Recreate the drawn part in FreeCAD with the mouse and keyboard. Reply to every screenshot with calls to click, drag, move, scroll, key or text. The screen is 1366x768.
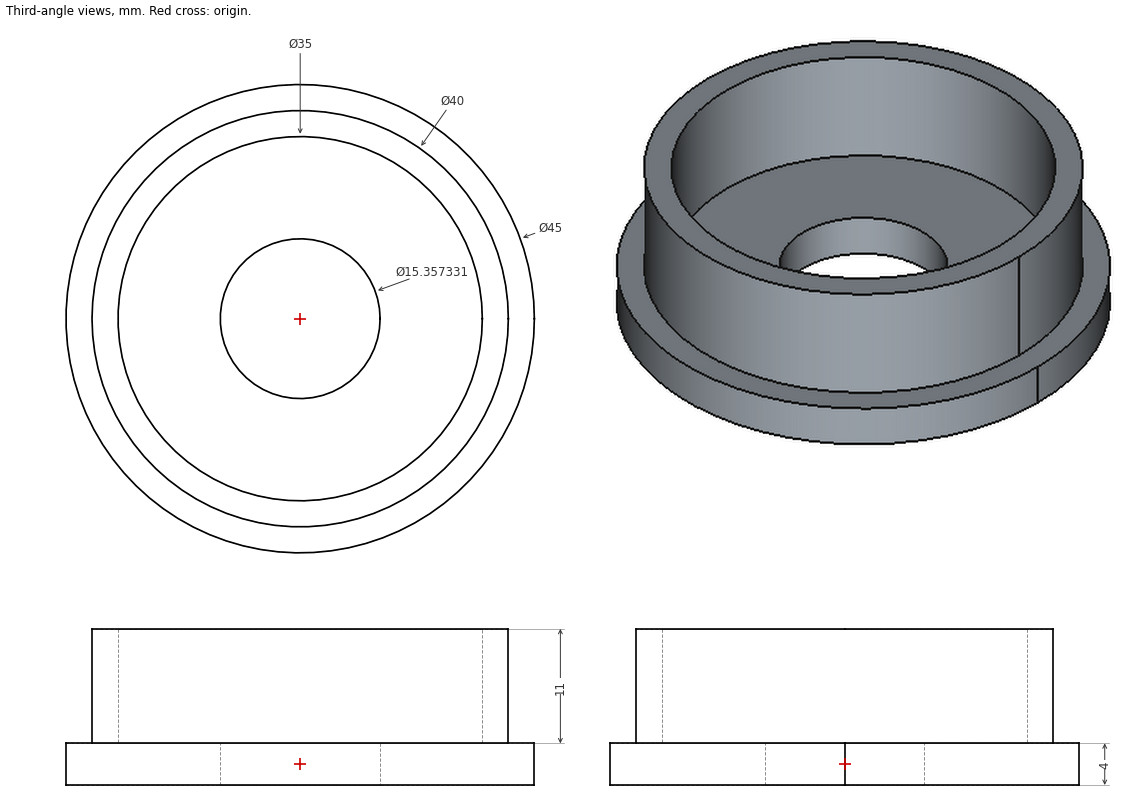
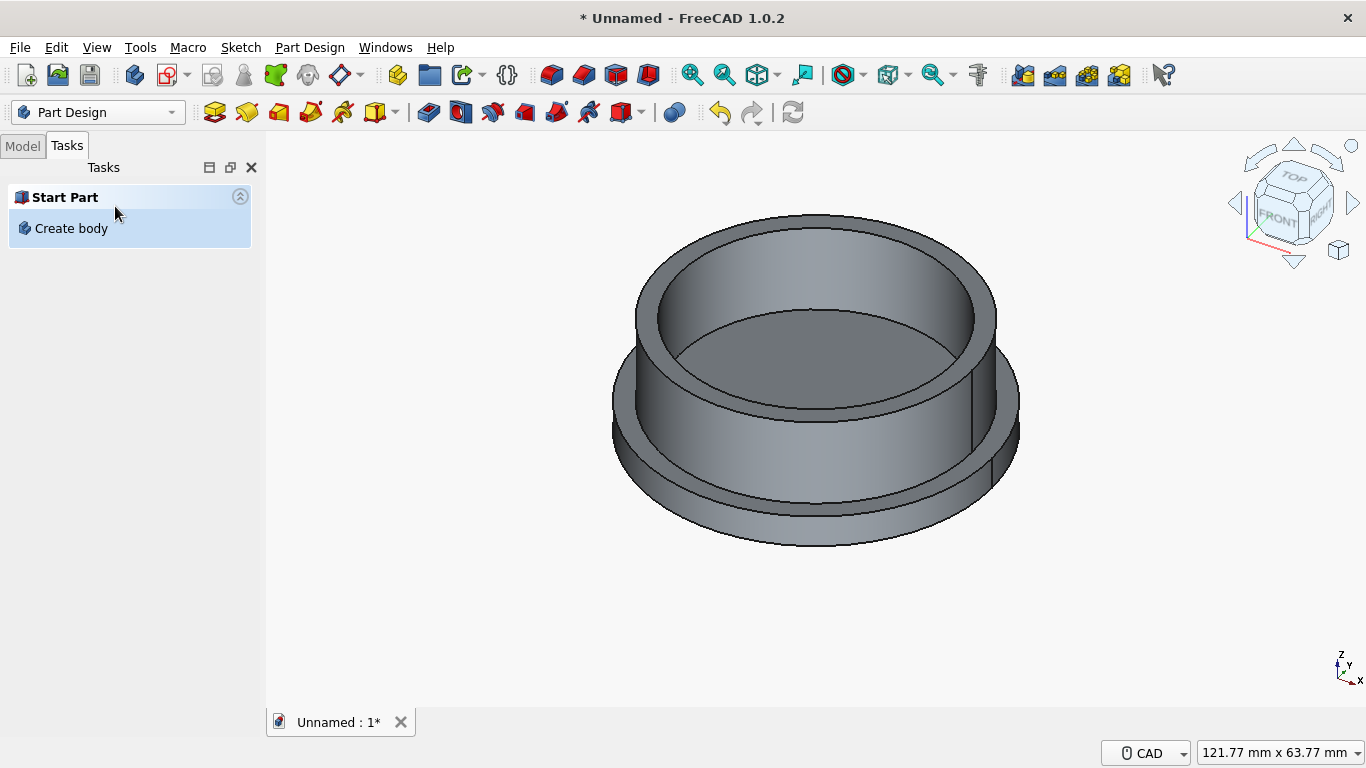
click(816, 399)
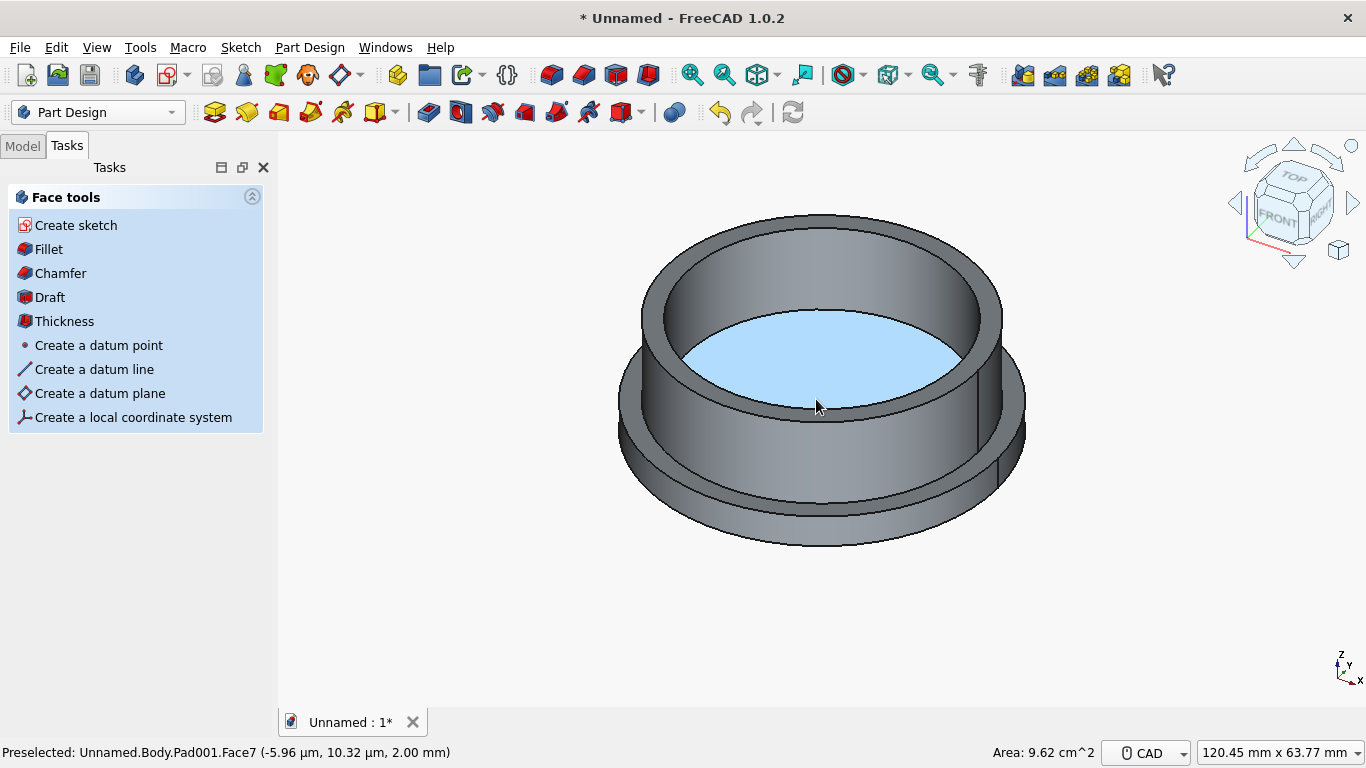
click(168, 76)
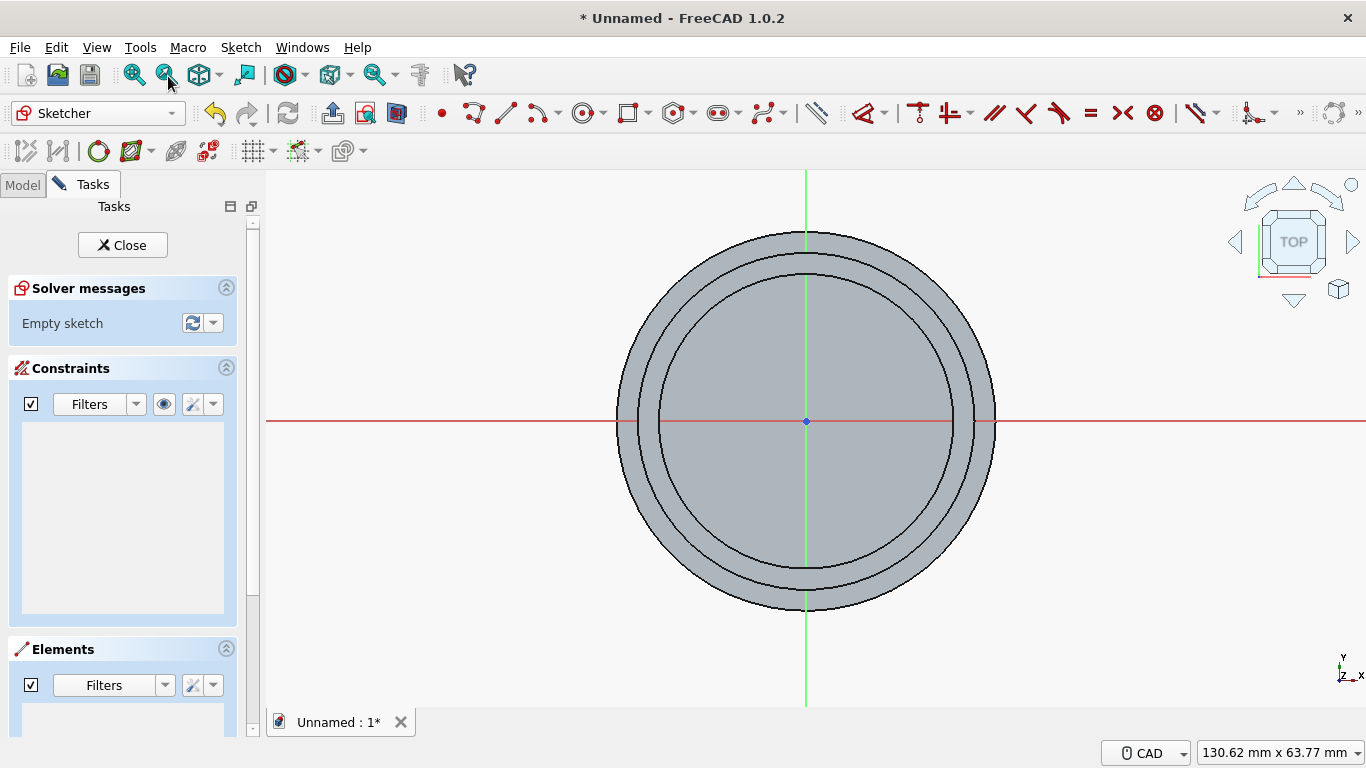
click(398, 114)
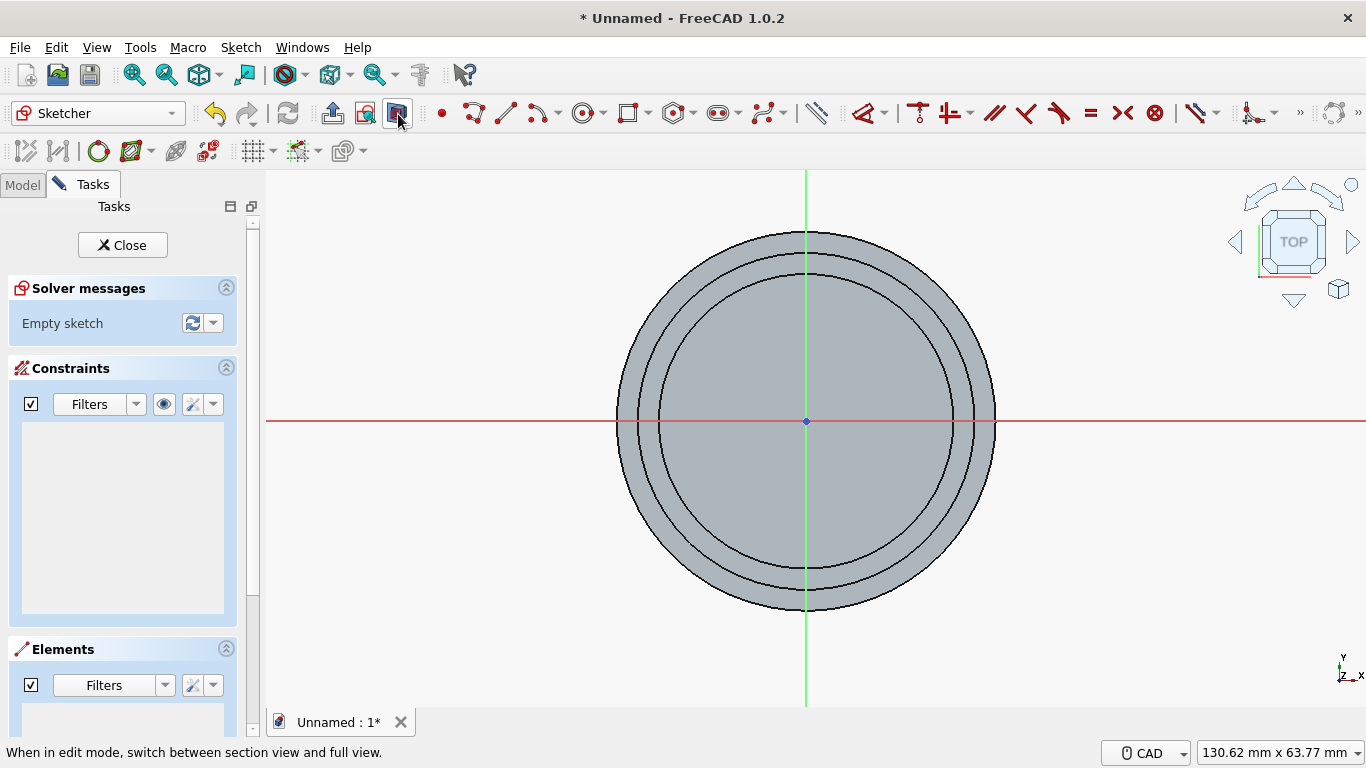
scroll(840, 411, up, 5)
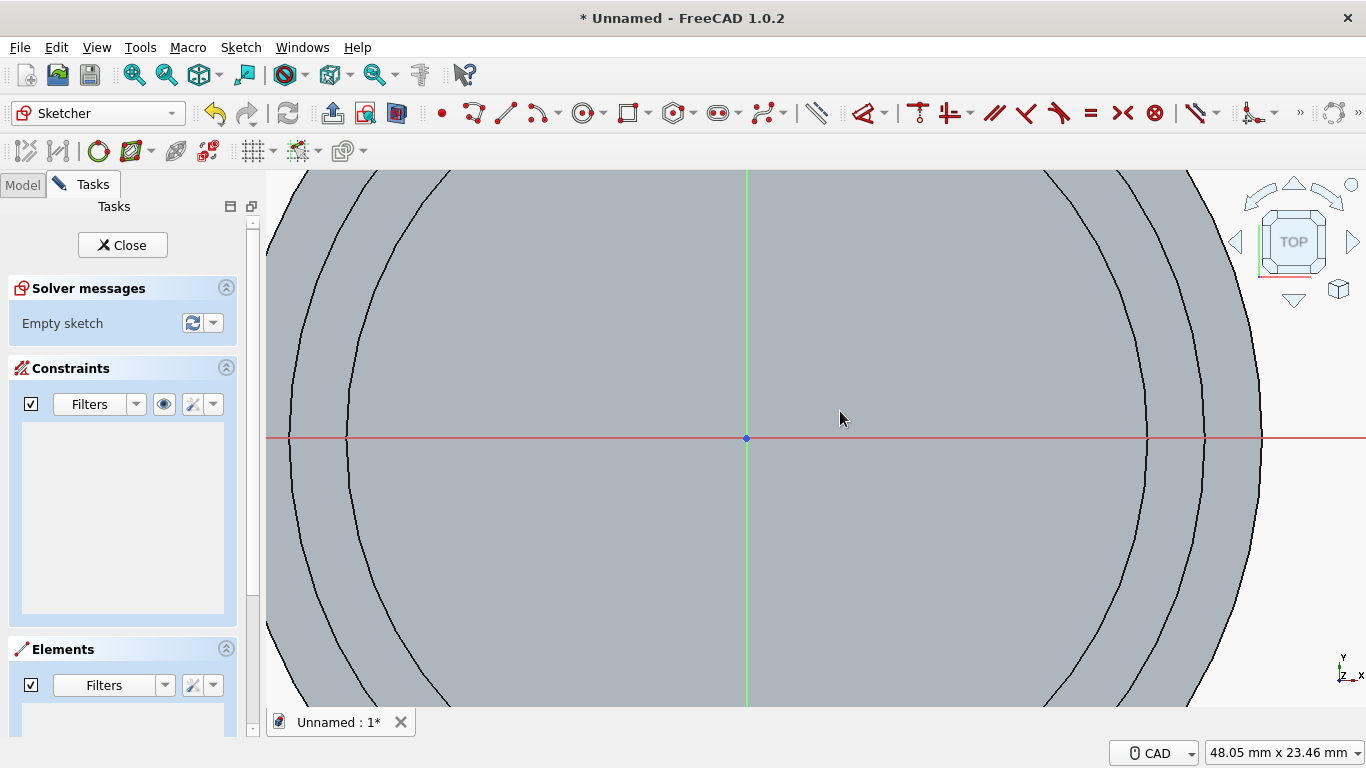
key(g)
key(c)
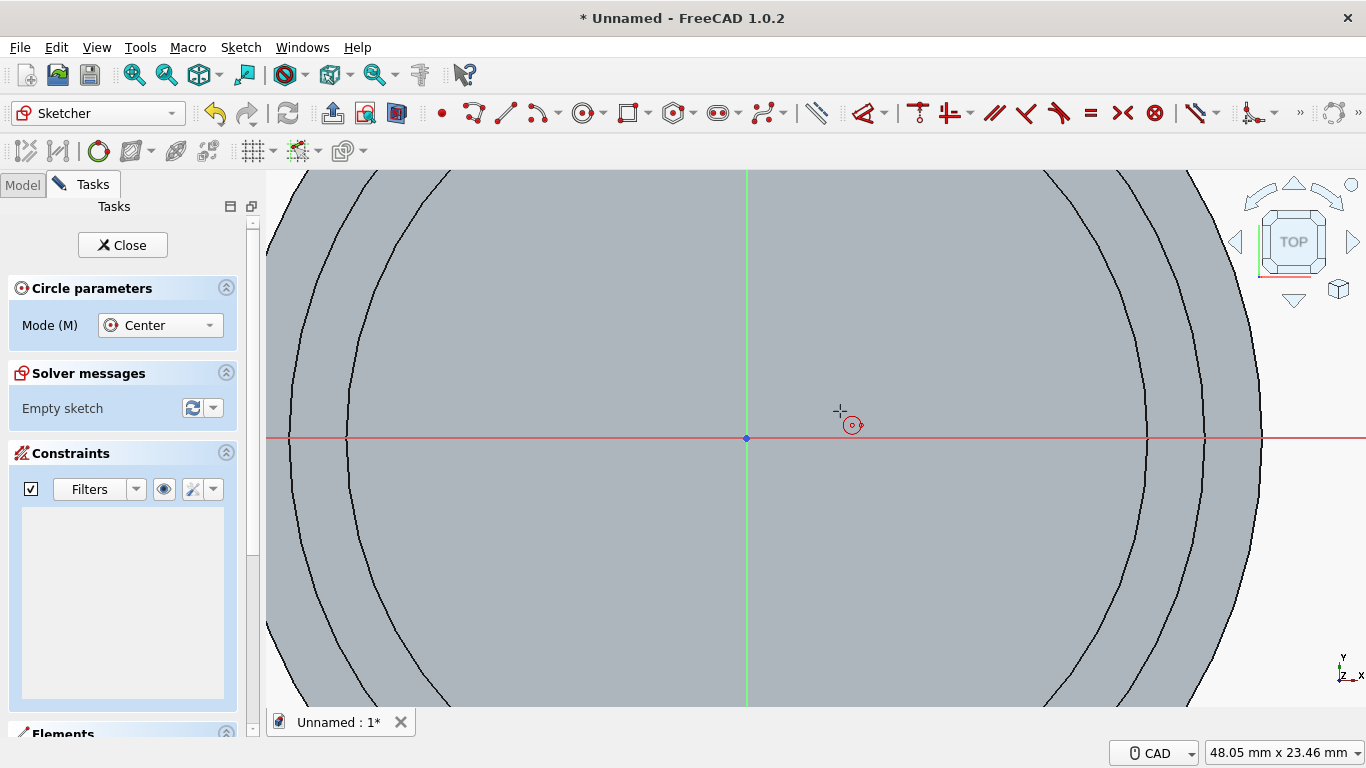
click(747, 438)
click(871, 314)
key(Escape)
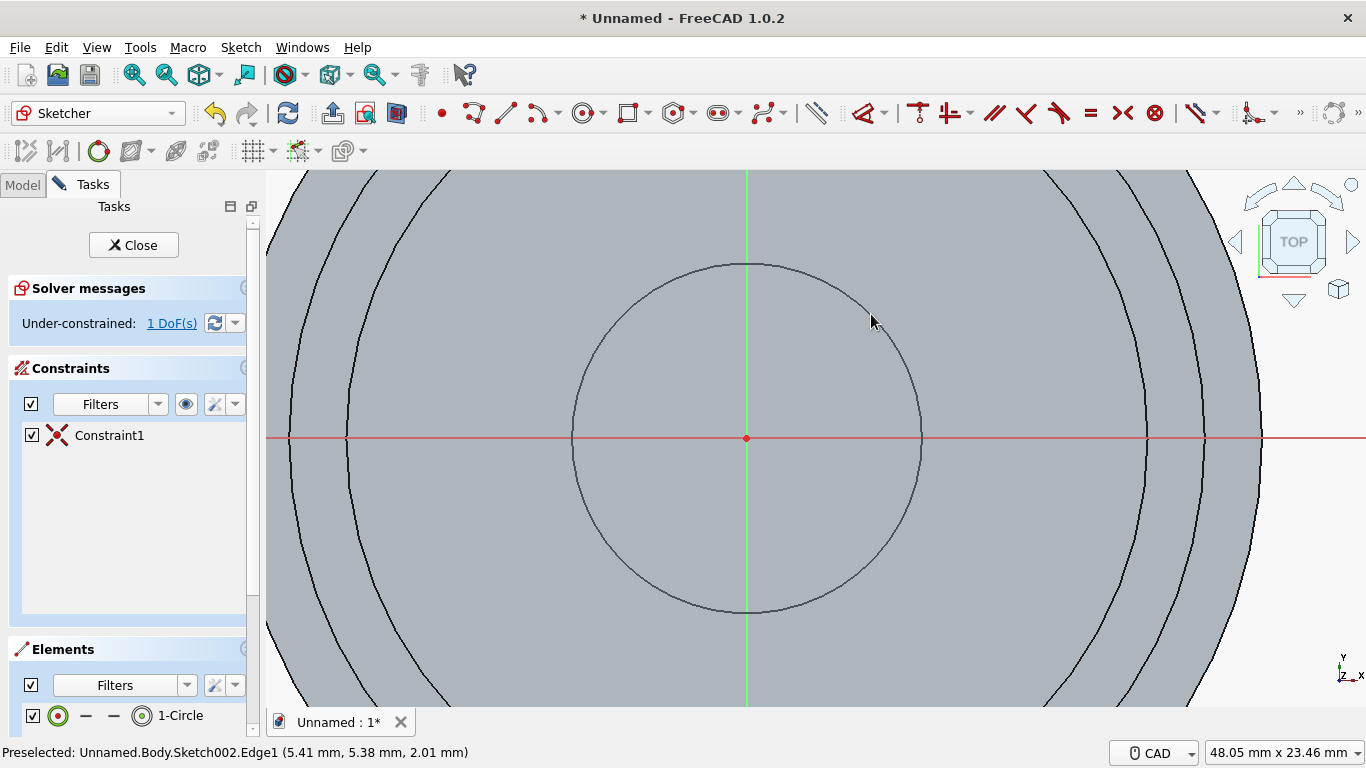
key(d)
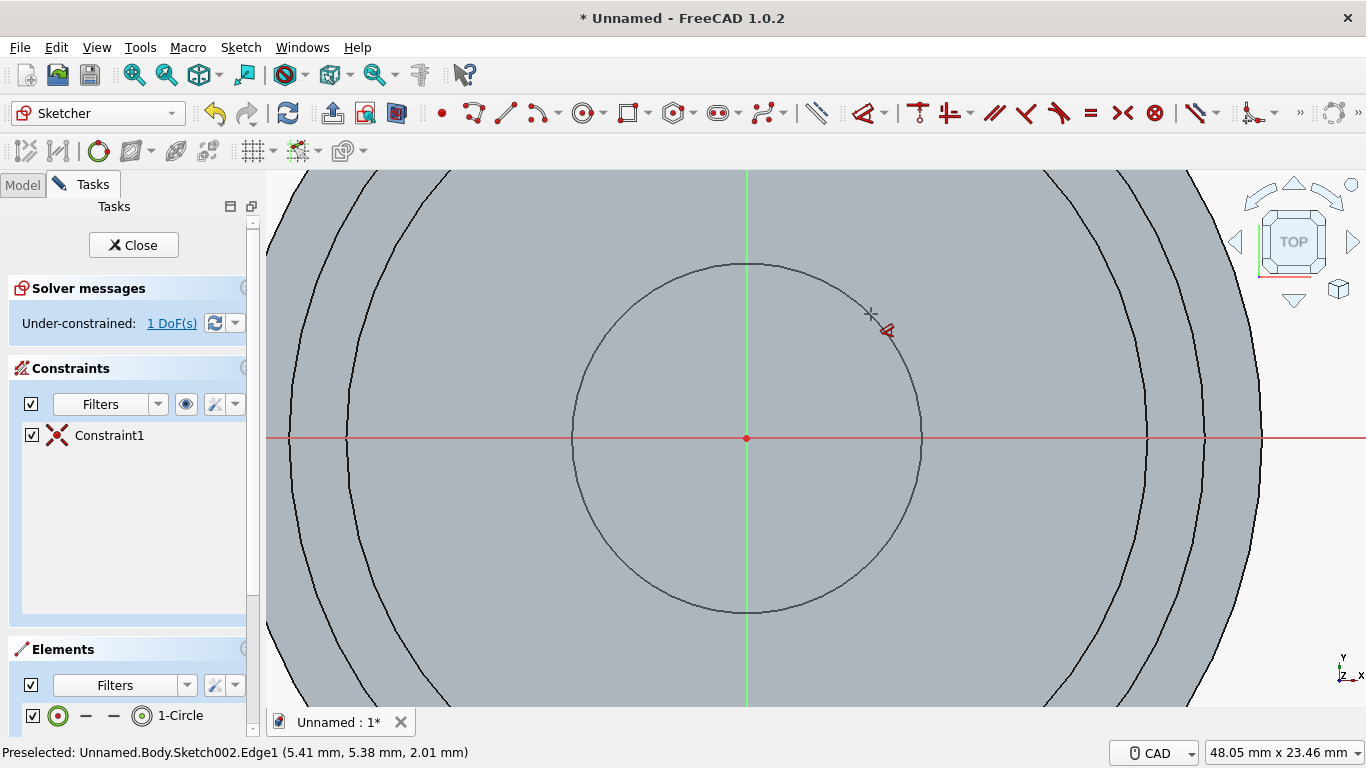
click(870, 314)
click(893, 291)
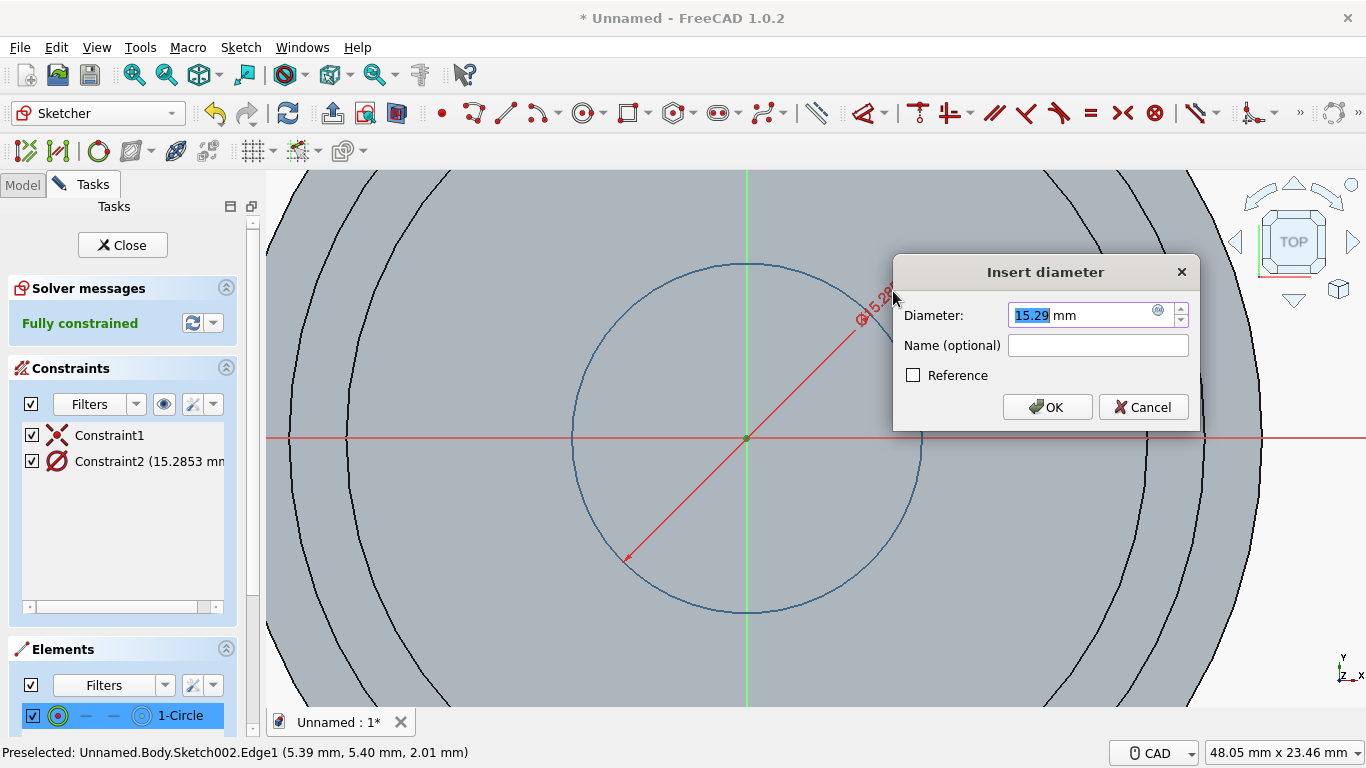
text(15.357331)
key(Return)
key(Escape)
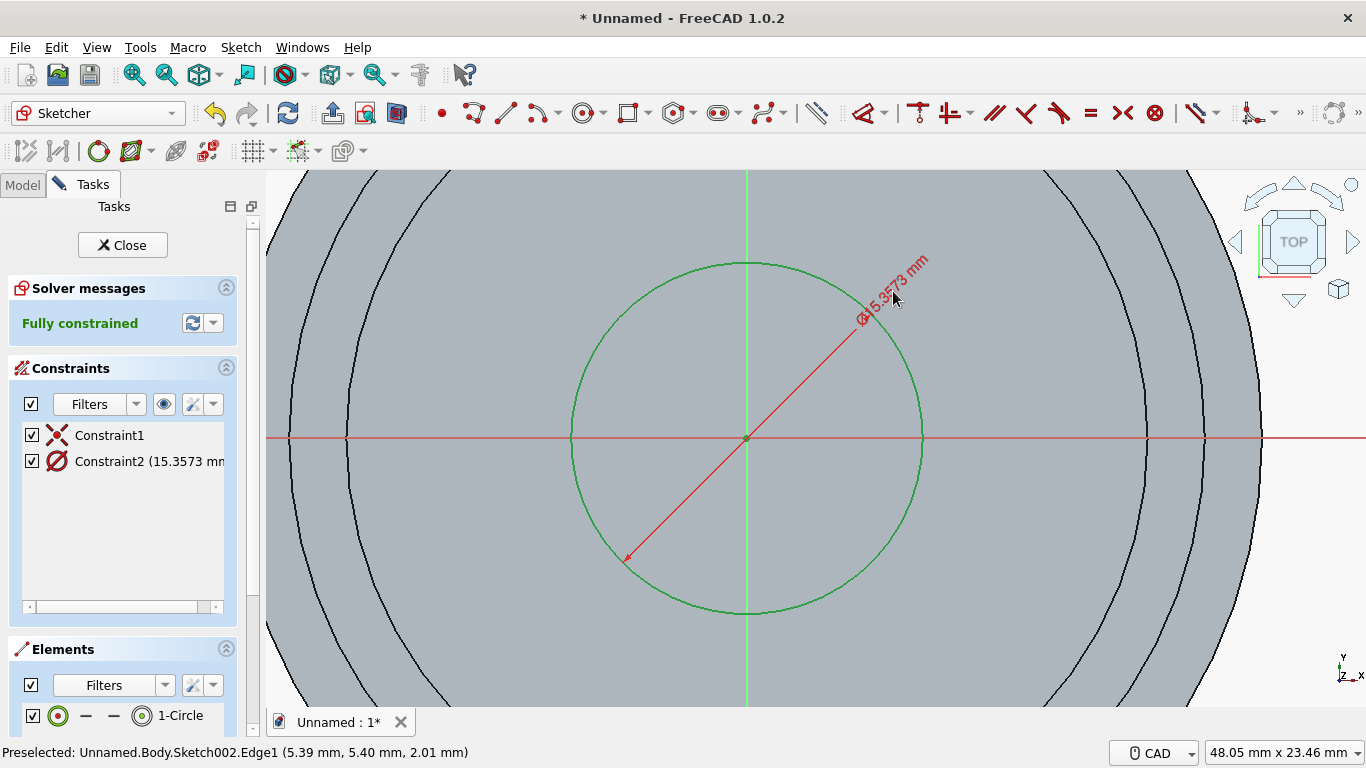
click(123, 245)